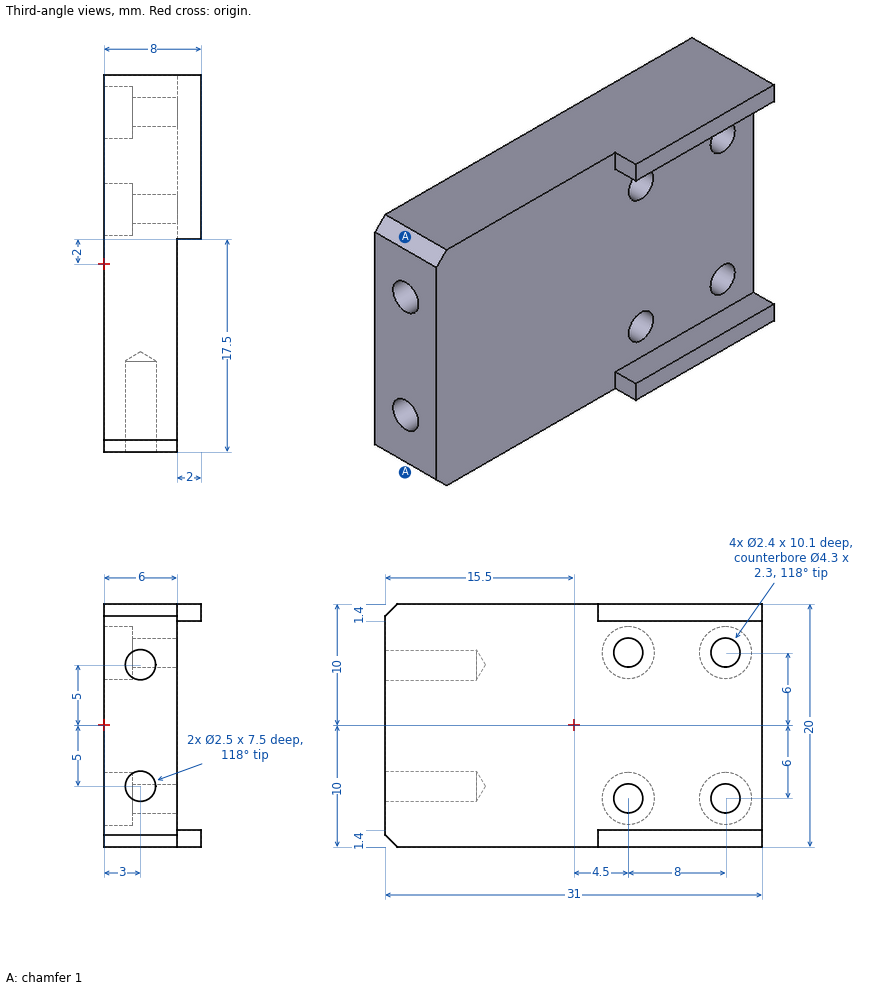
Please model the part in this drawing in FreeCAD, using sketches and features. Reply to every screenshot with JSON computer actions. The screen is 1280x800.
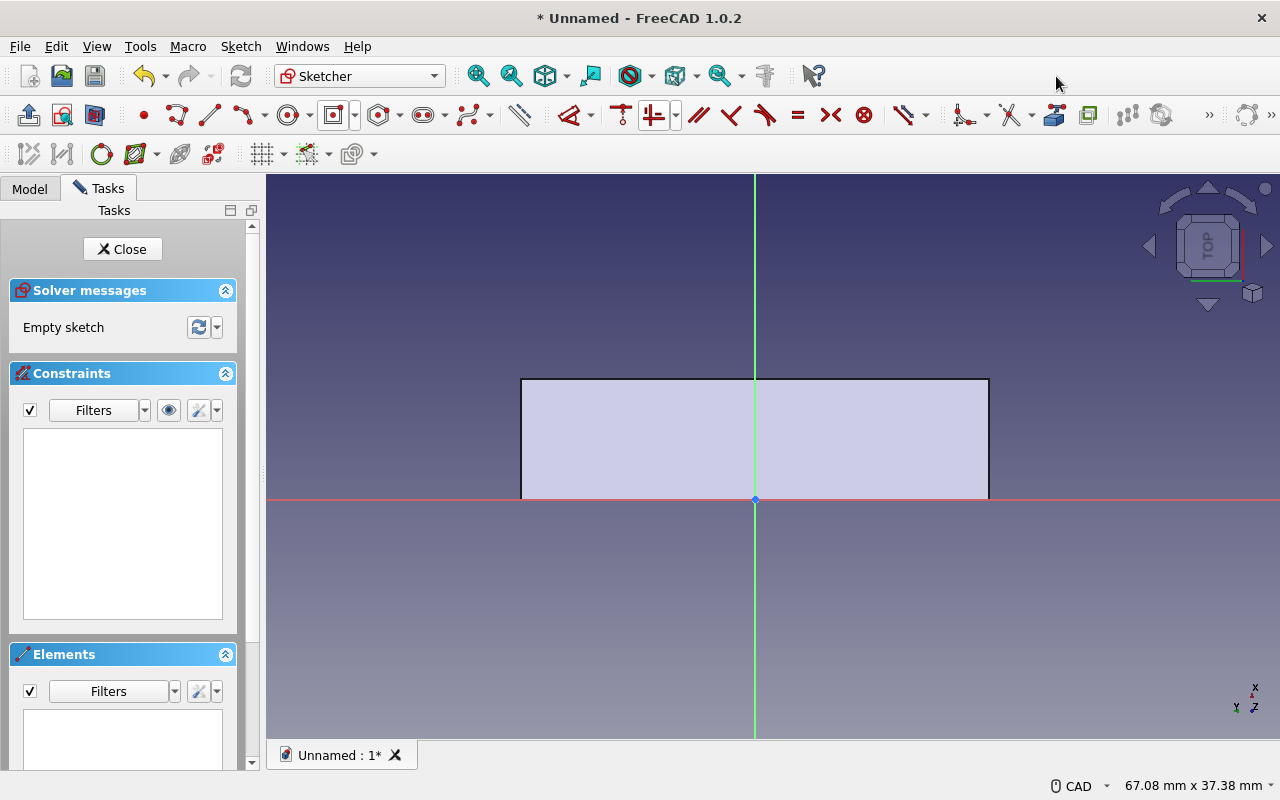
{"action": "scroll", "coordinate": [982, 425], "scroll_direction": "up", "scroll_amount": 4}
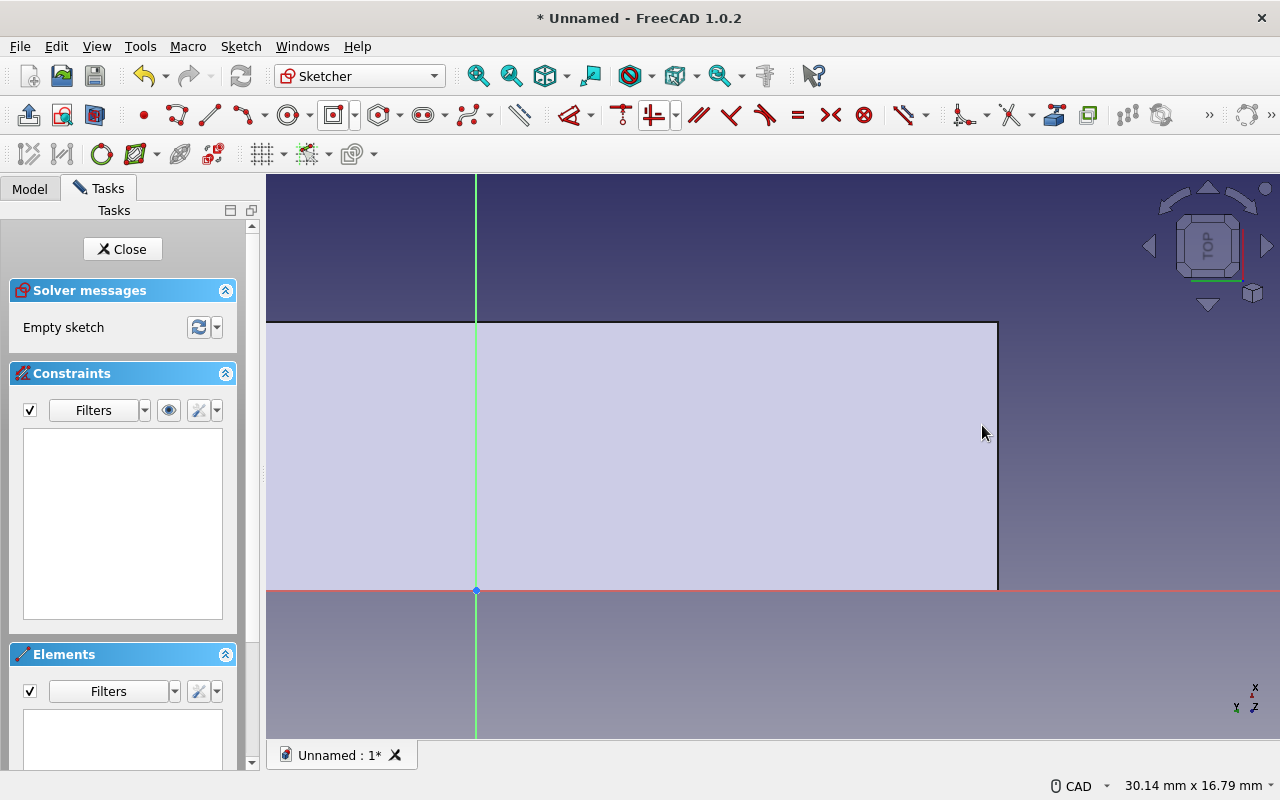
{"action": "left_click", "coordinate": [354, 116]}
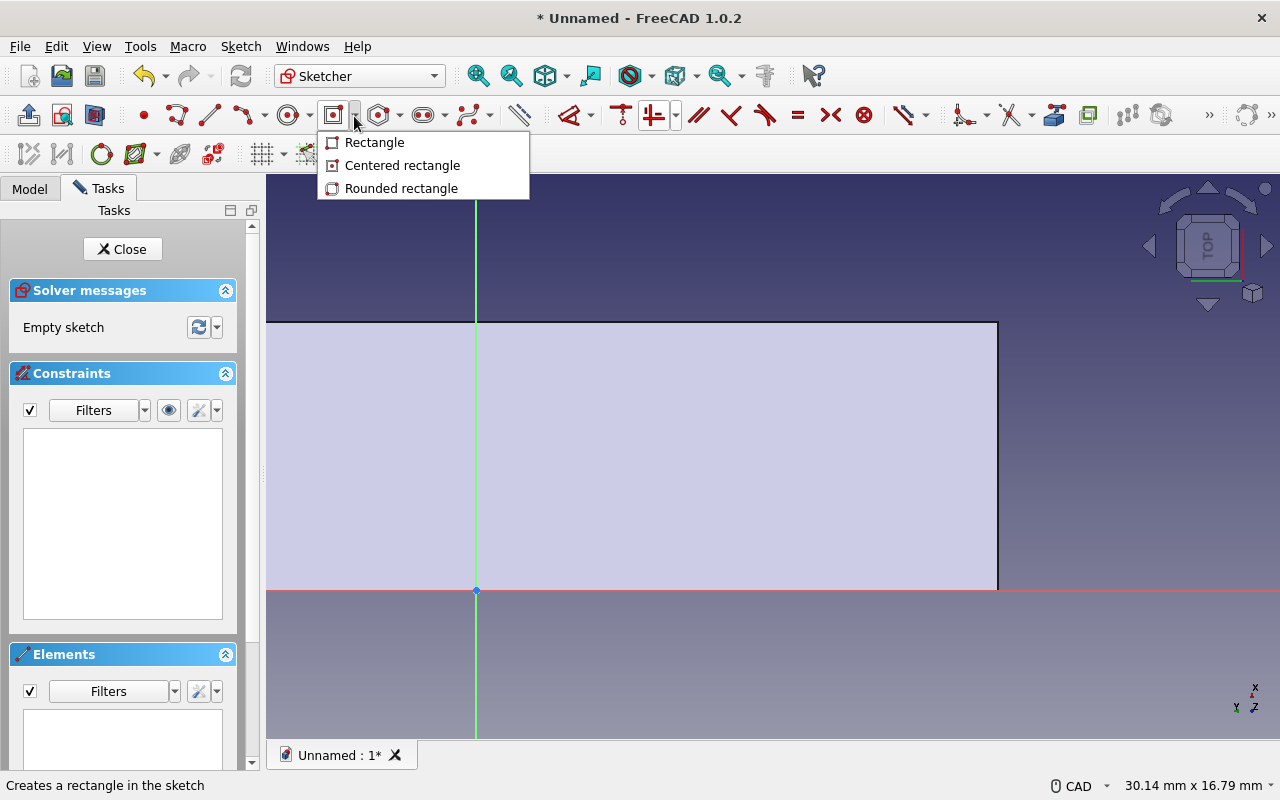
{"action": "left_click", "coordinate": [424, 142]}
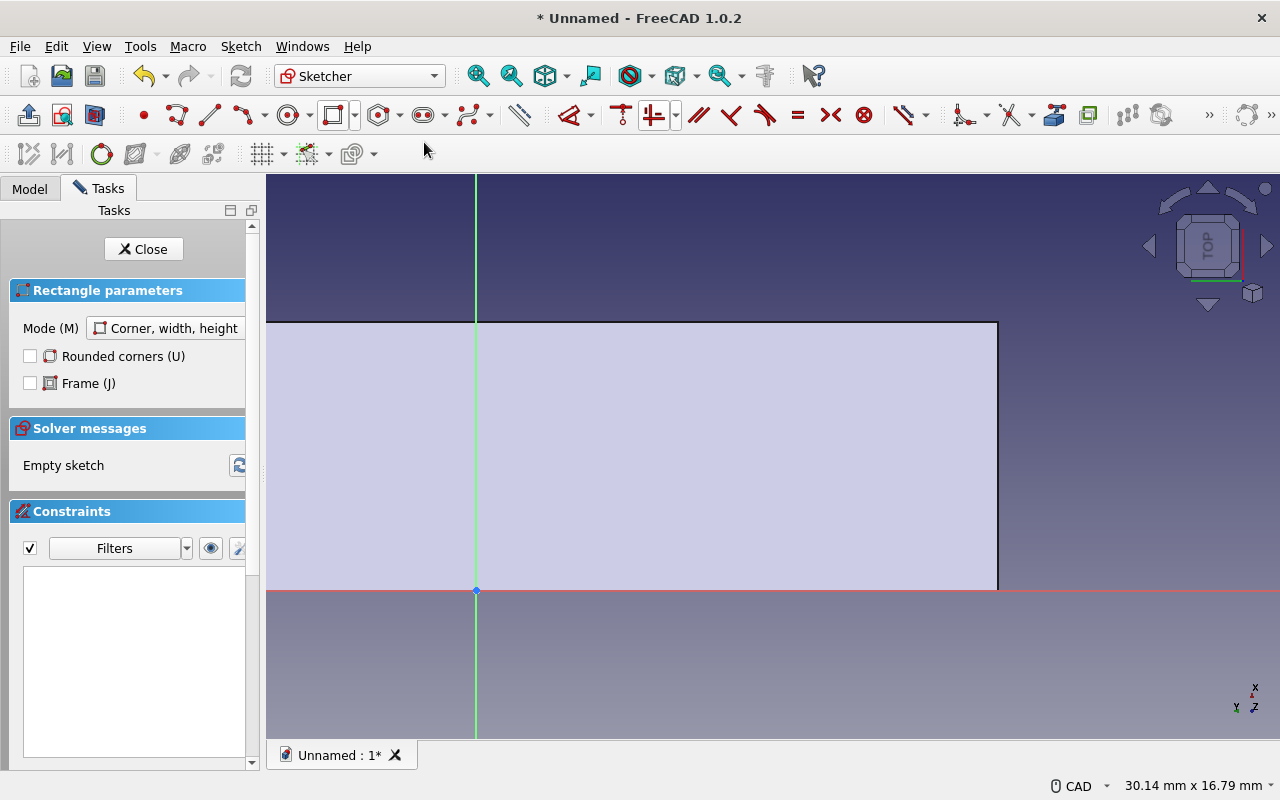
{"action": "left_click", "coordinate": [409, 322]}
{"action": "left_click", "coordinate": [998, 389]}
{"action": "key", "text": "Escape"}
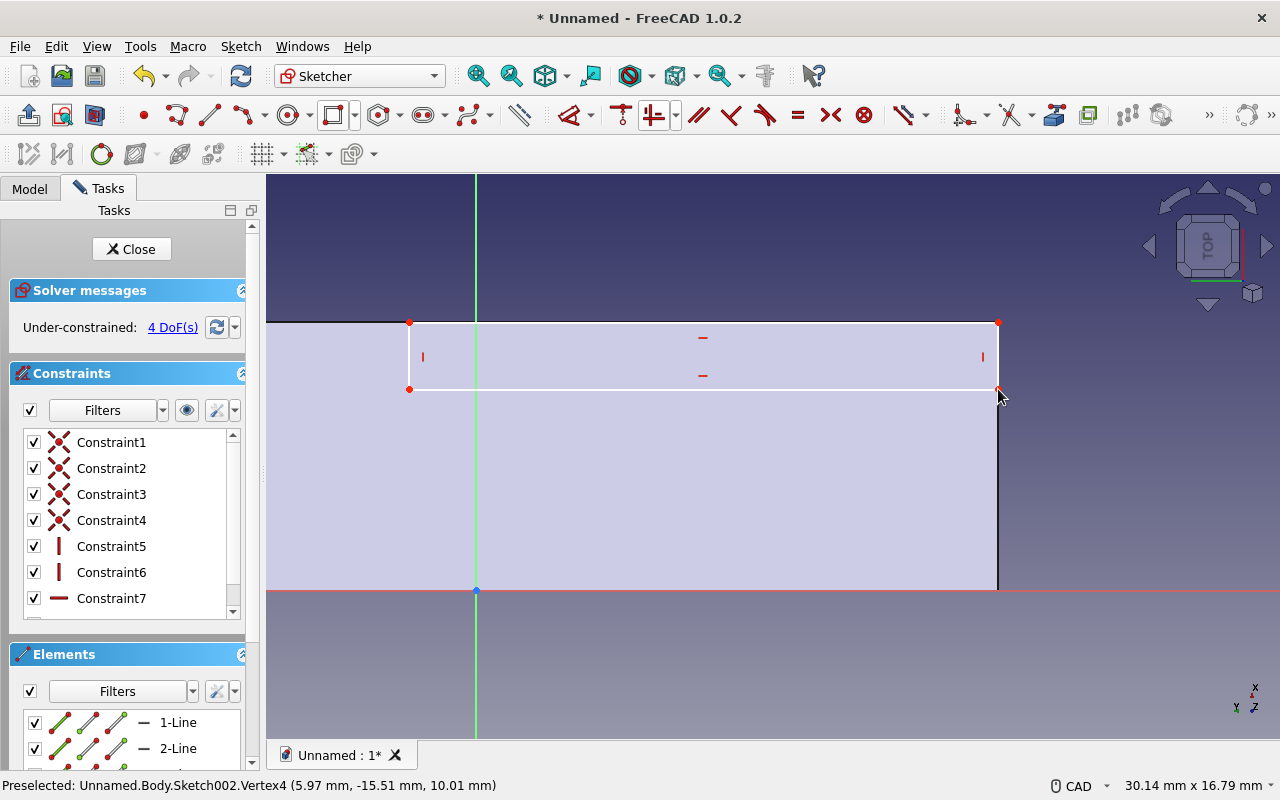
{"action": "left_click", "coordinate": [568, 116]}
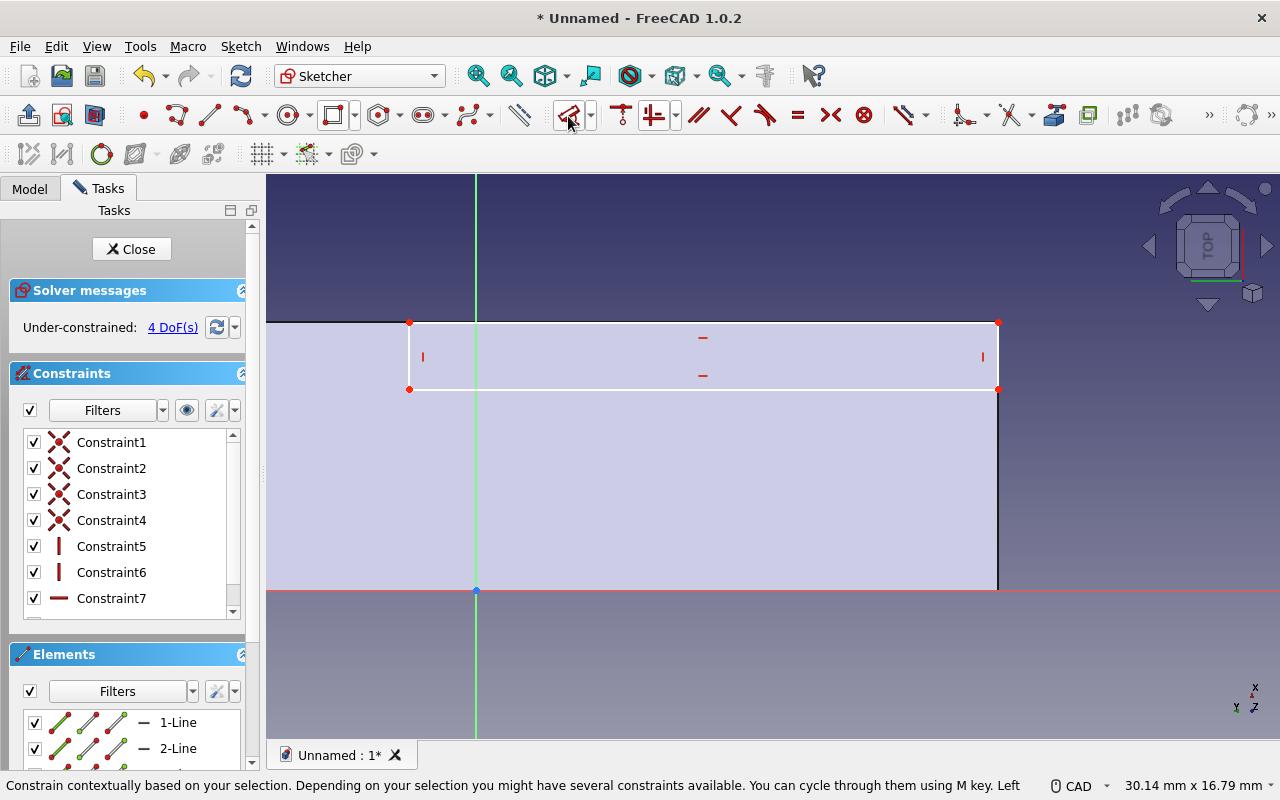
{"action": "left_click", "coordinate": [409, 343]}
{"action": "left_click", "coordinate": [375, 357]}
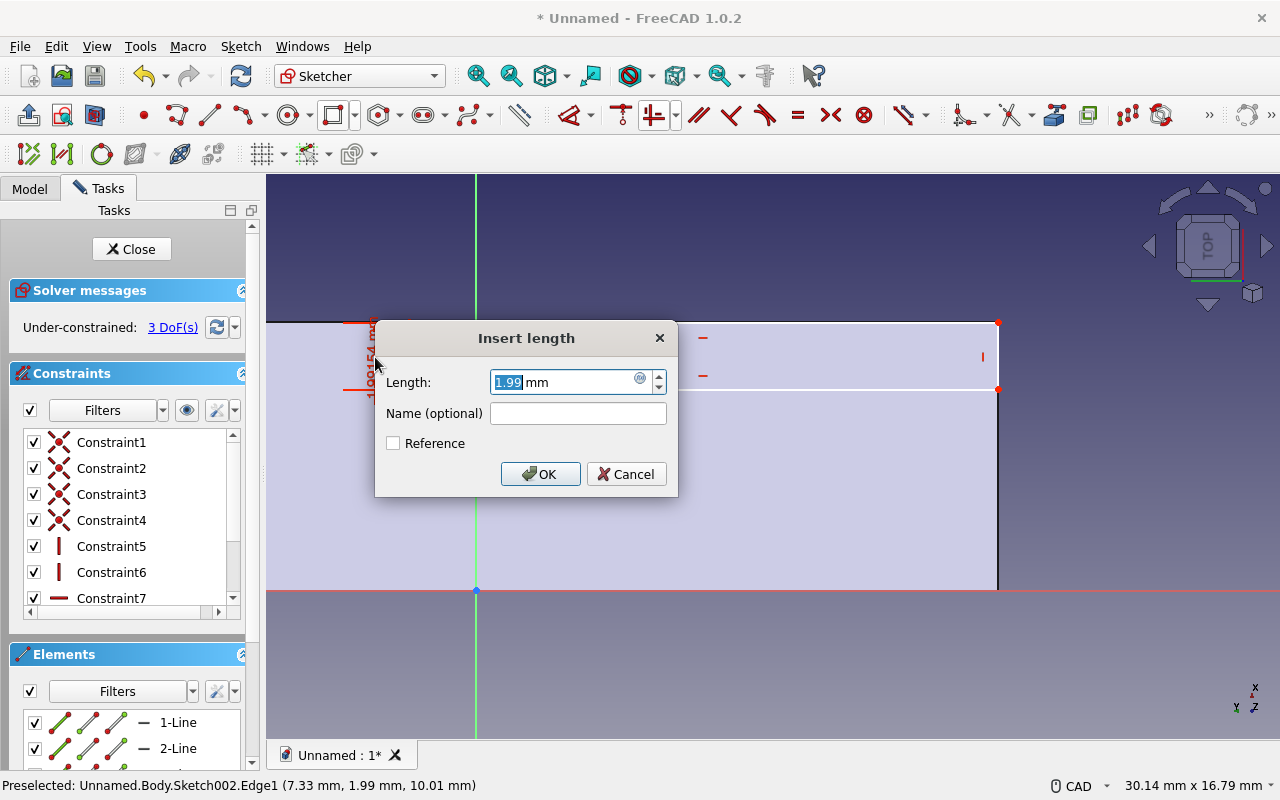
{"action": "type", "text": "2"}
{"action": "key", "text": "Return"}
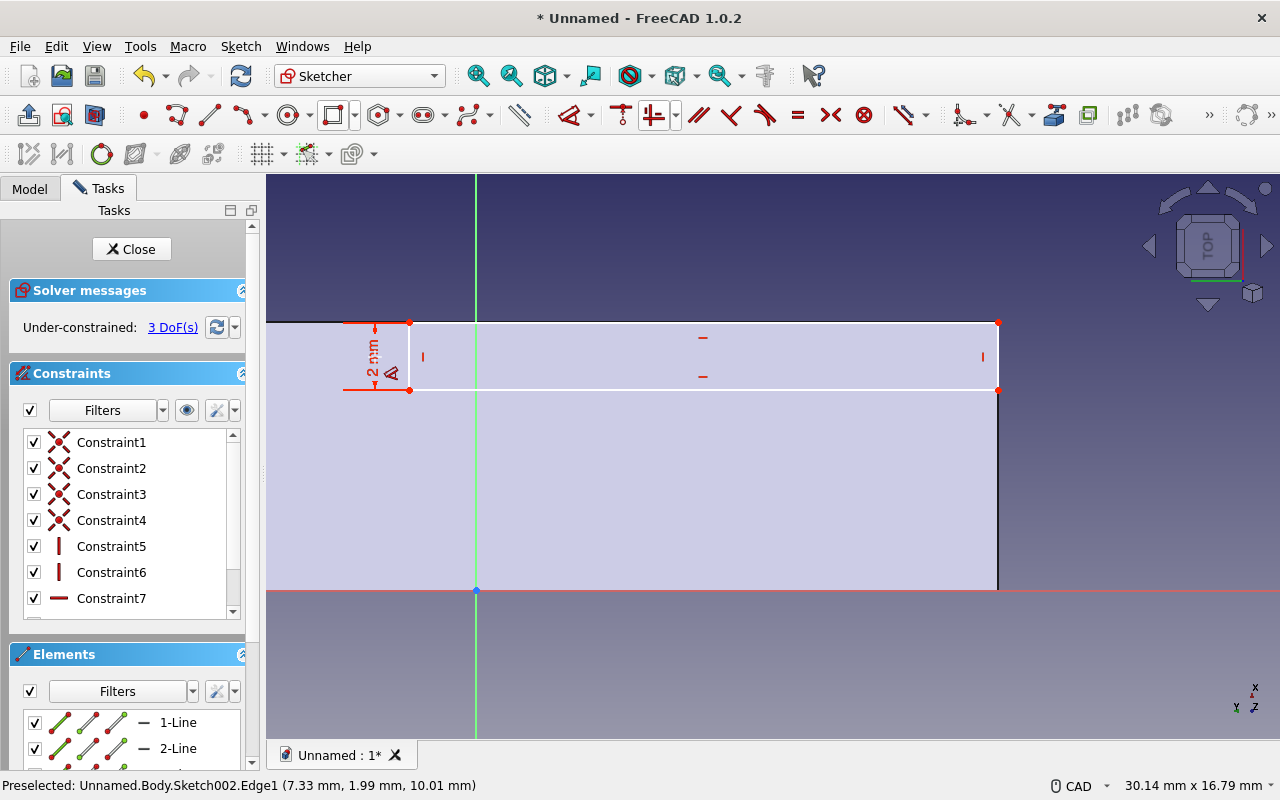
{"action": "left_click", "coordinate": [409, 323]}
{"action": "left_click", "coordinate": [443, 625]}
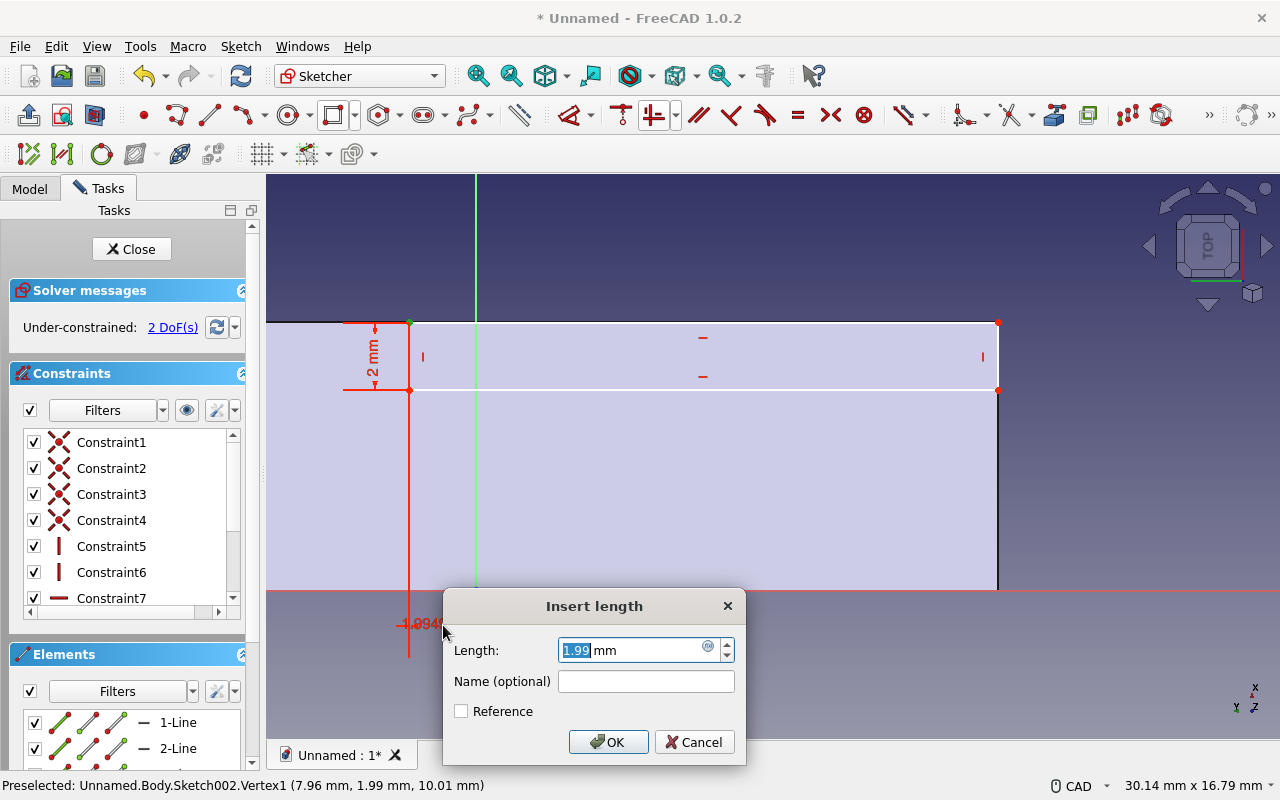
{"action": "type", "text": "2"}
{"action": "key", "text": "Return"}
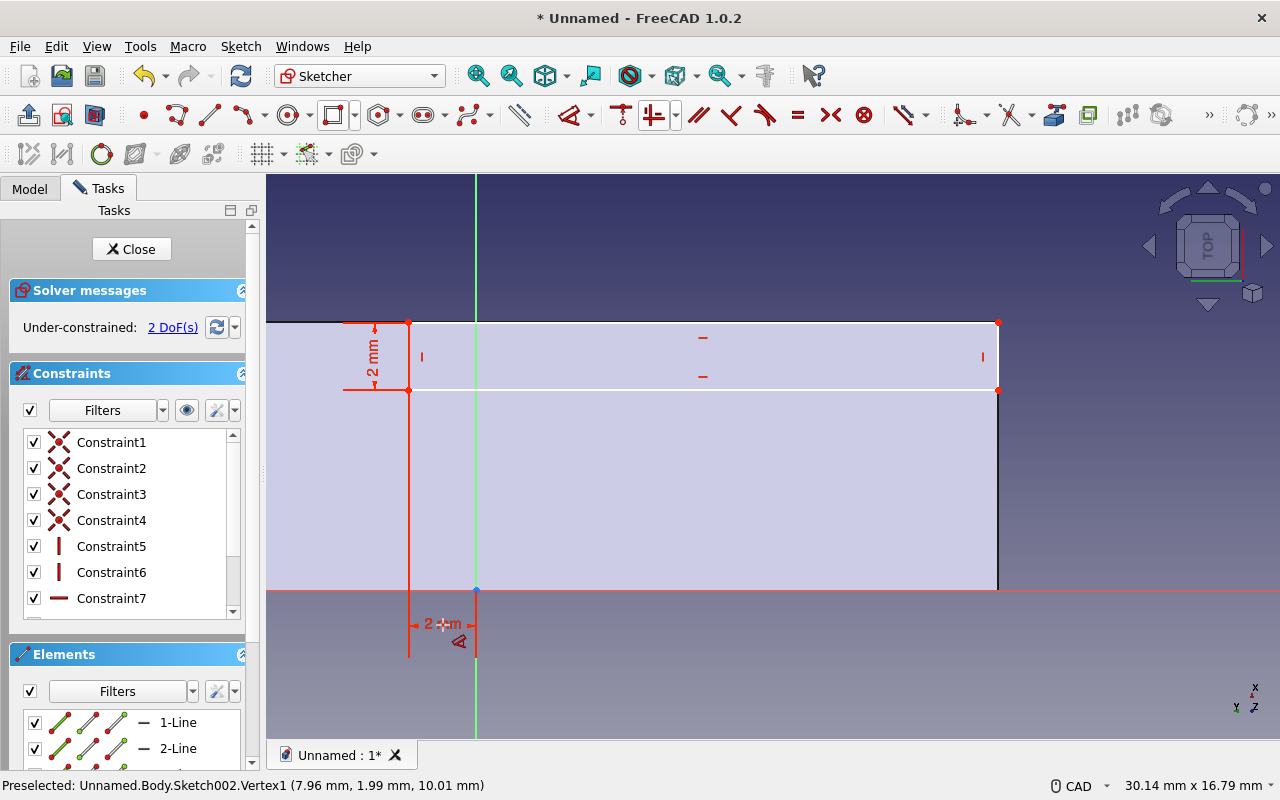
{"action": "left_click", "coordinate": [409, 323]}
{"action": "left_click", "coordinate": [375, 457]}